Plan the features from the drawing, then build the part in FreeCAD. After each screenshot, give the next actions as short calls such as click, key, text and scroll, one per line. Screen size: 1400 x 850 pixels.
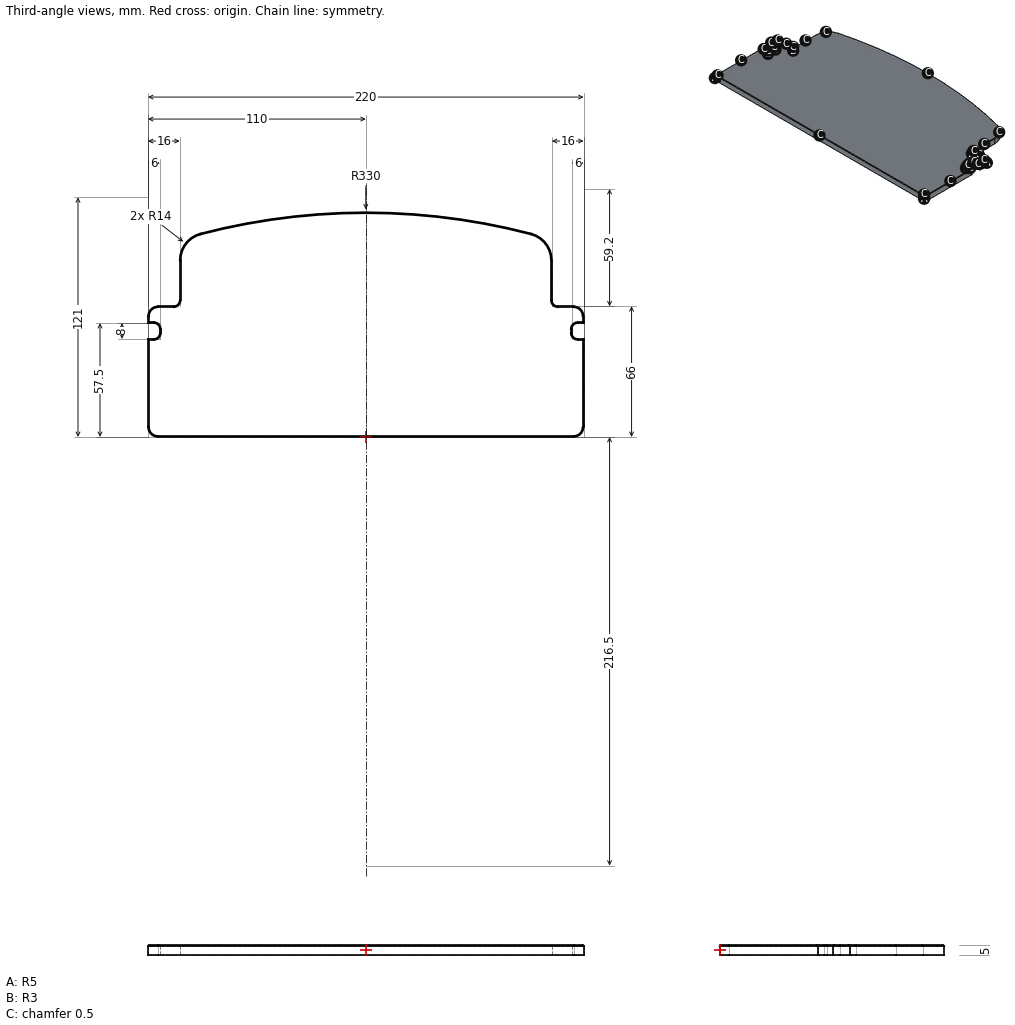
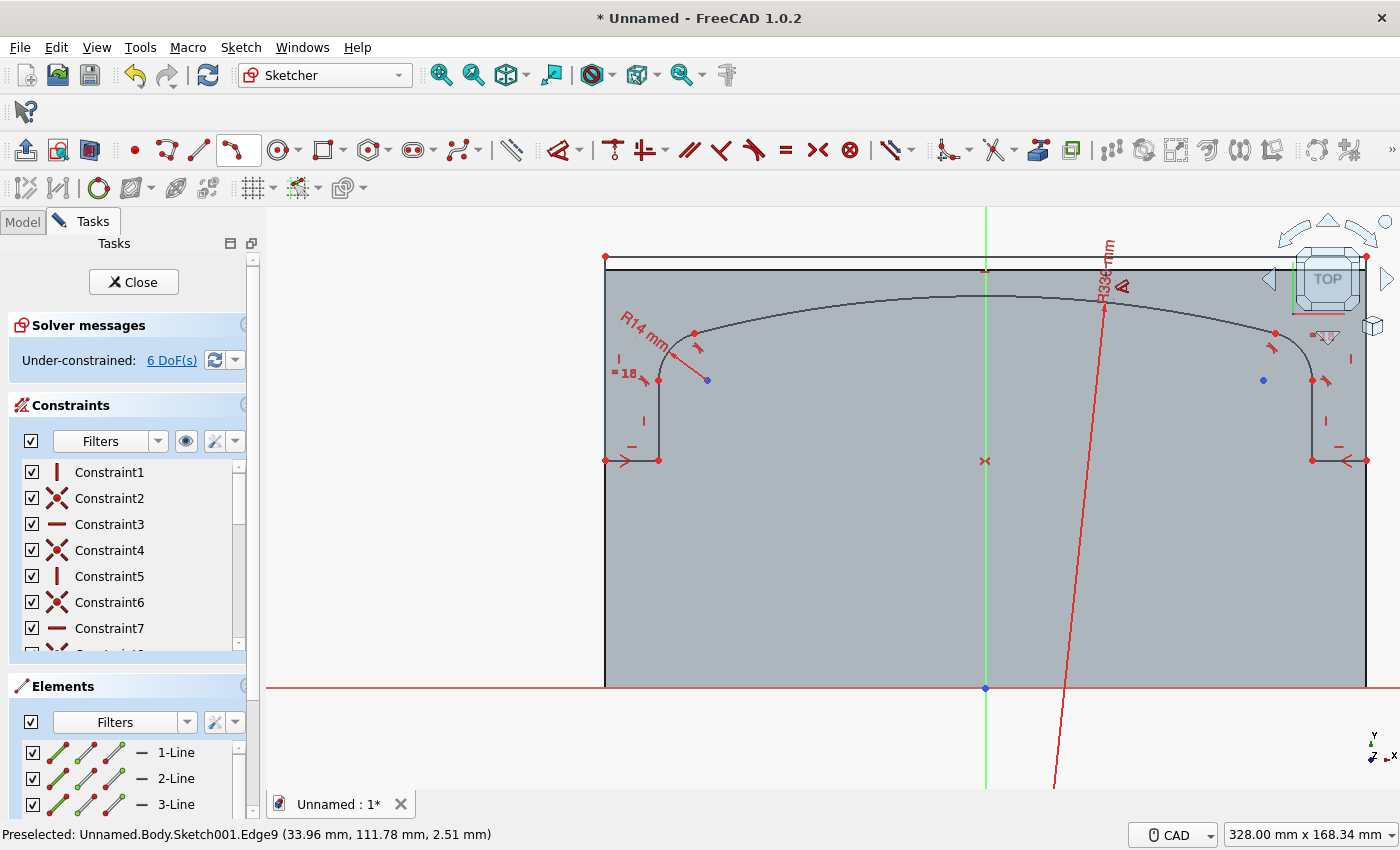
scroll(294, 617, down, 1)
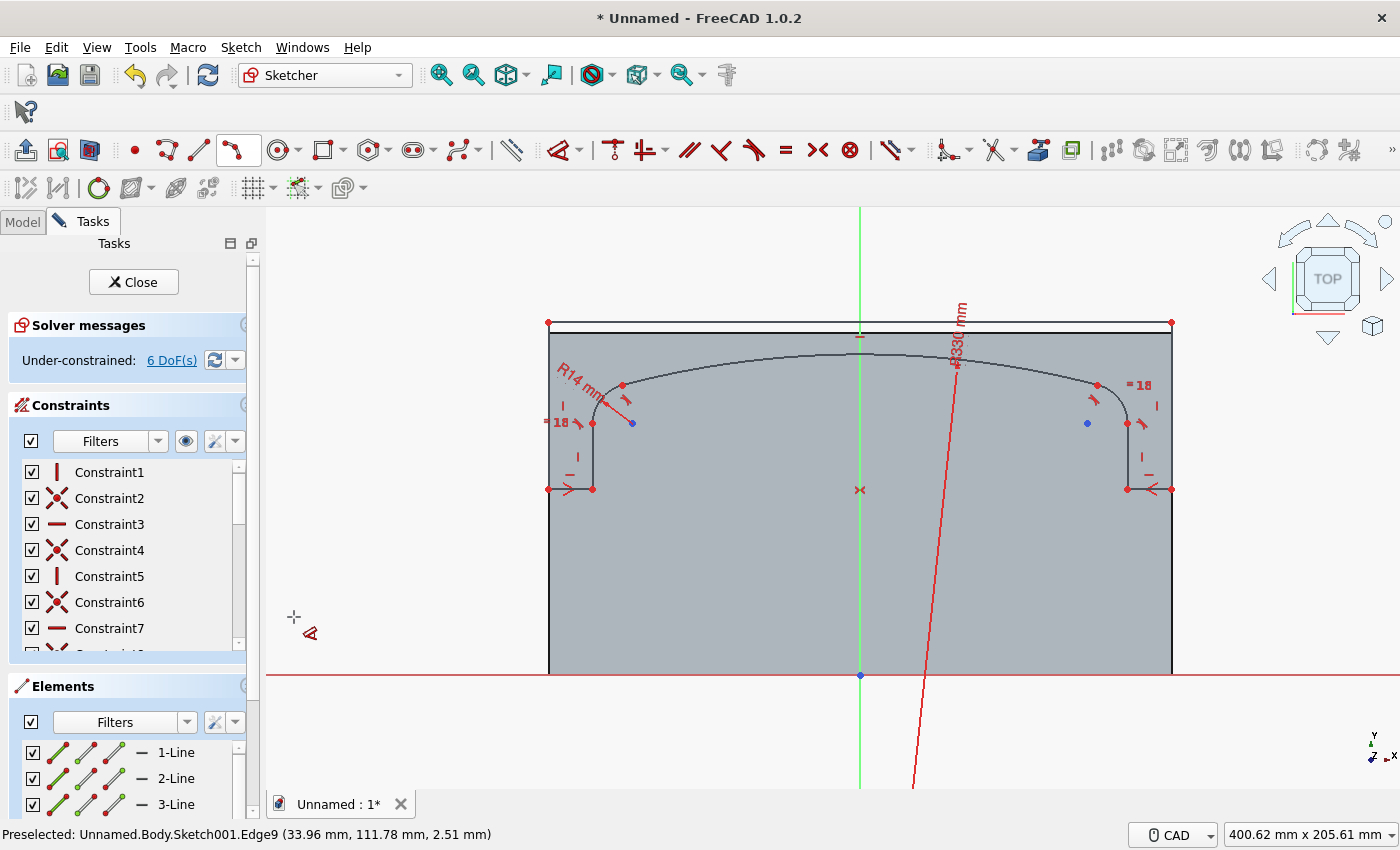
click(1141, 489)
click(1150, 455)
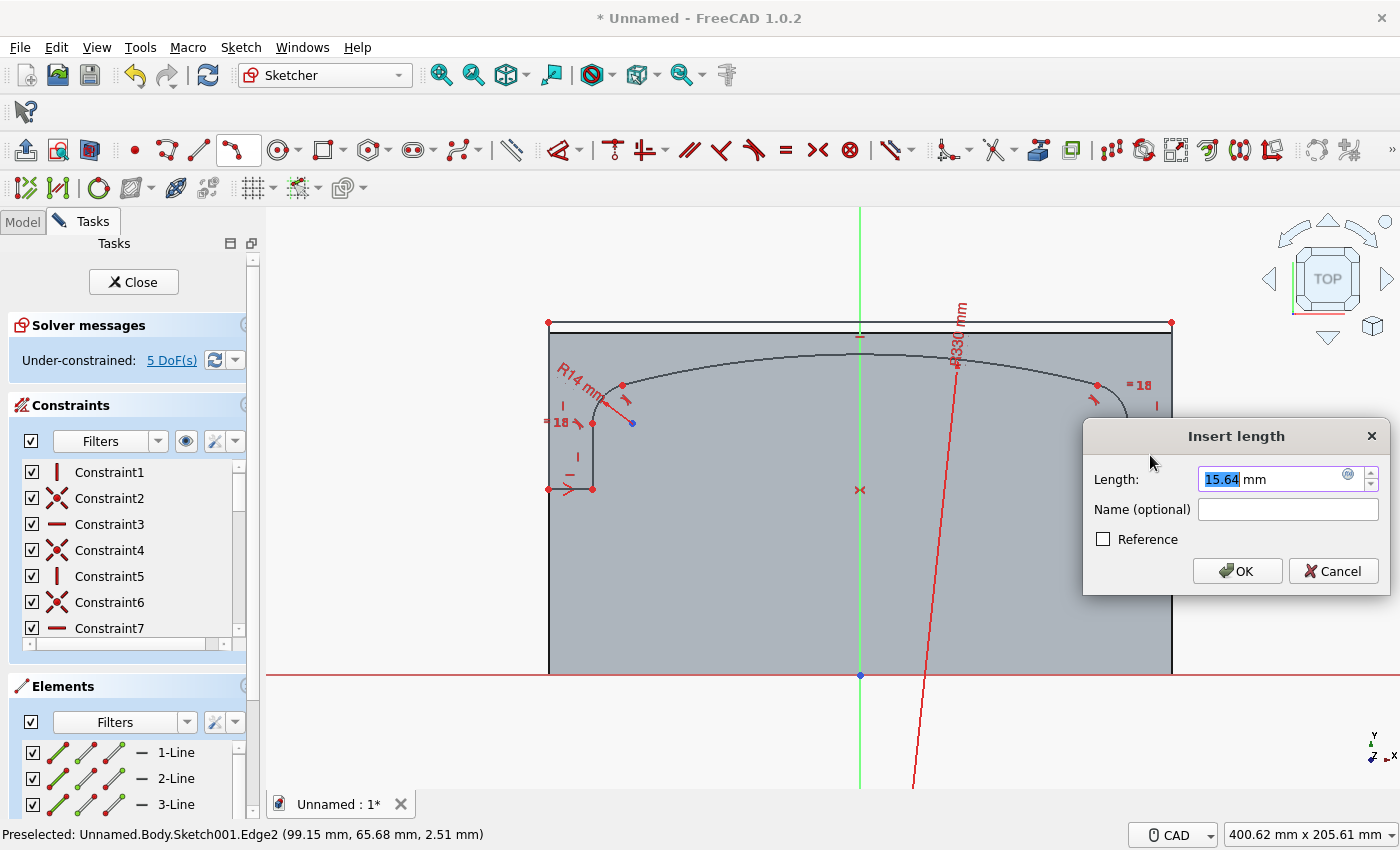
text(16)
key(Return)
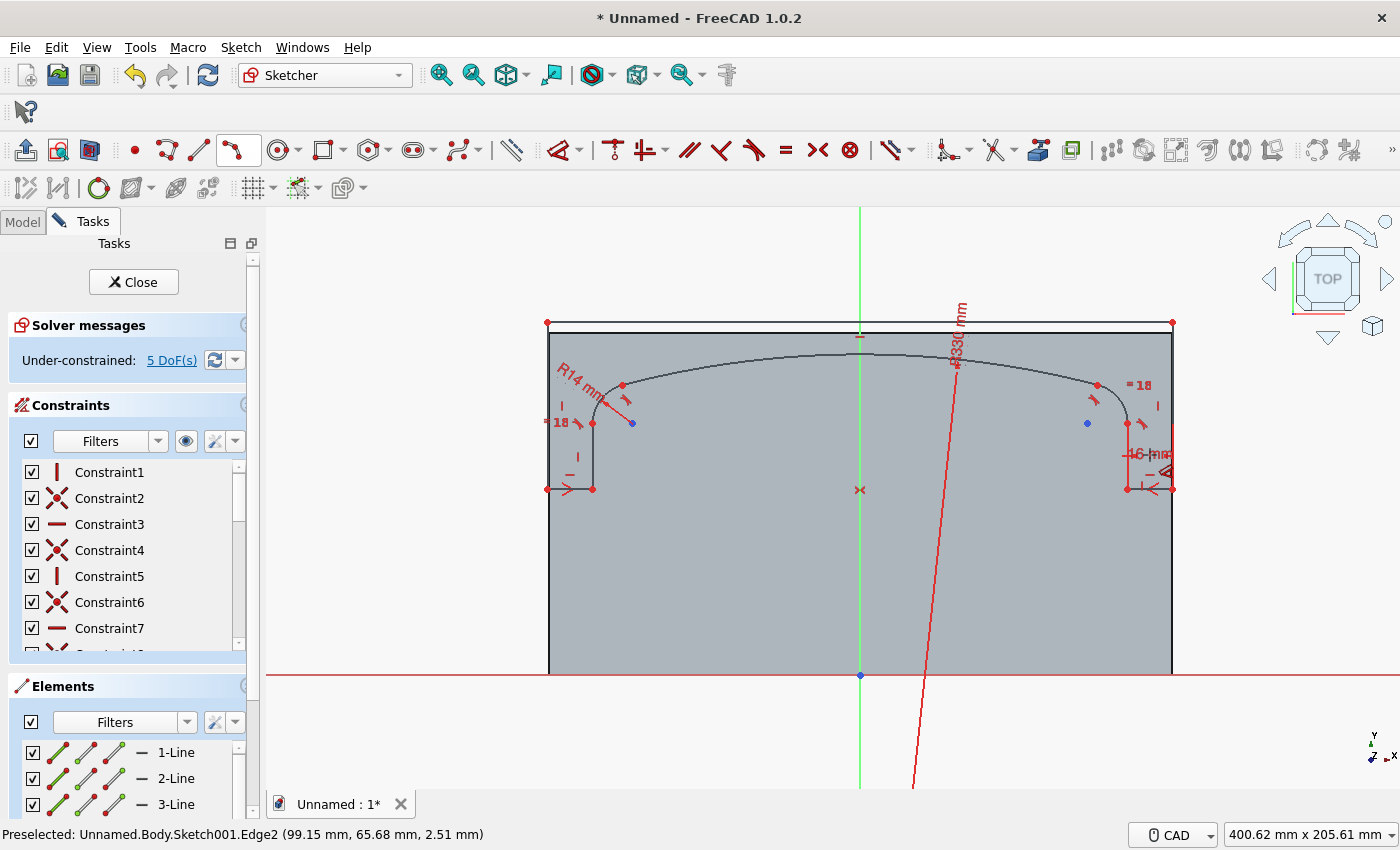
click(561, 489)
click(570, 455)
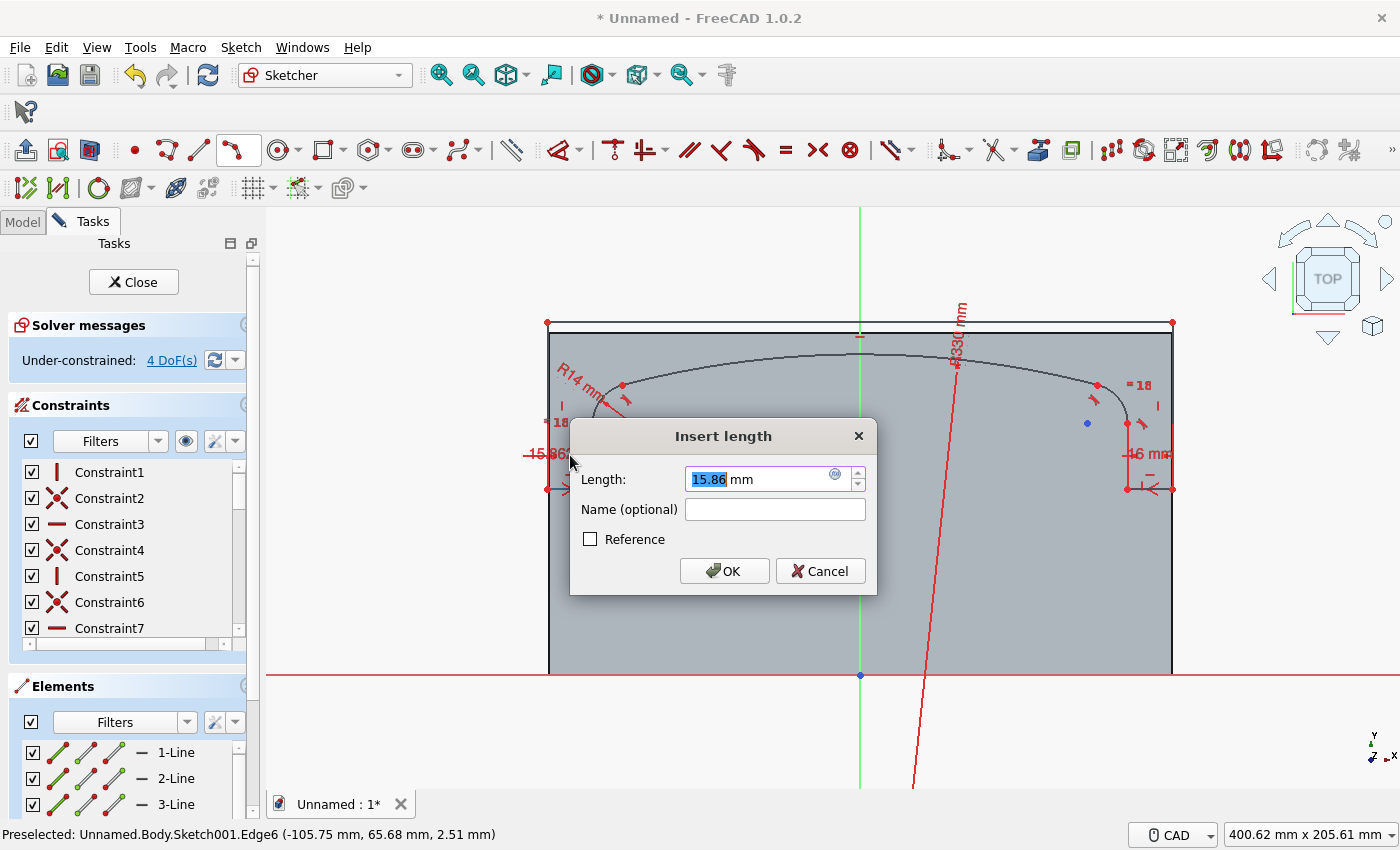
text(16)
key(Return)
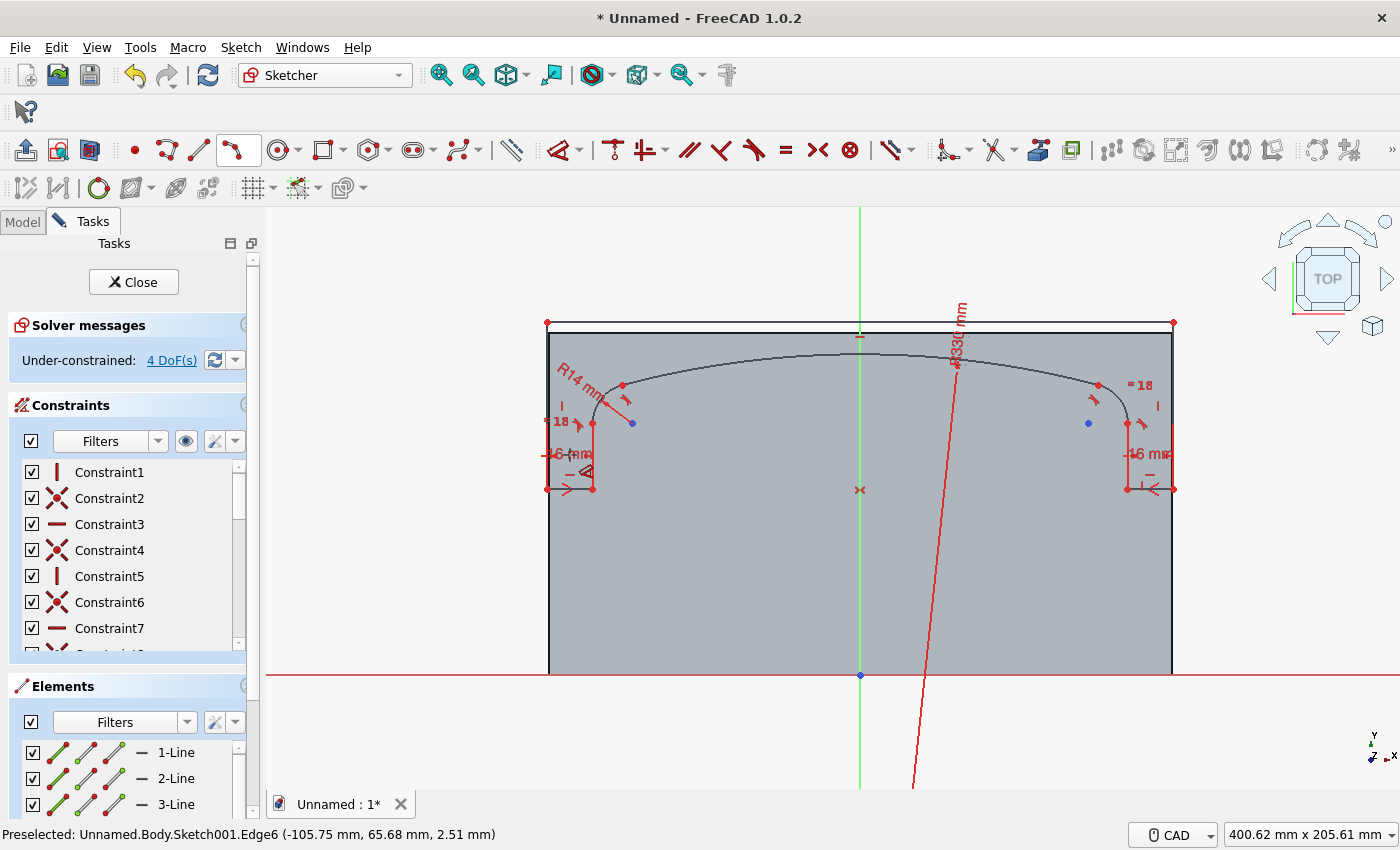
click(985, 322)
click(716, 288)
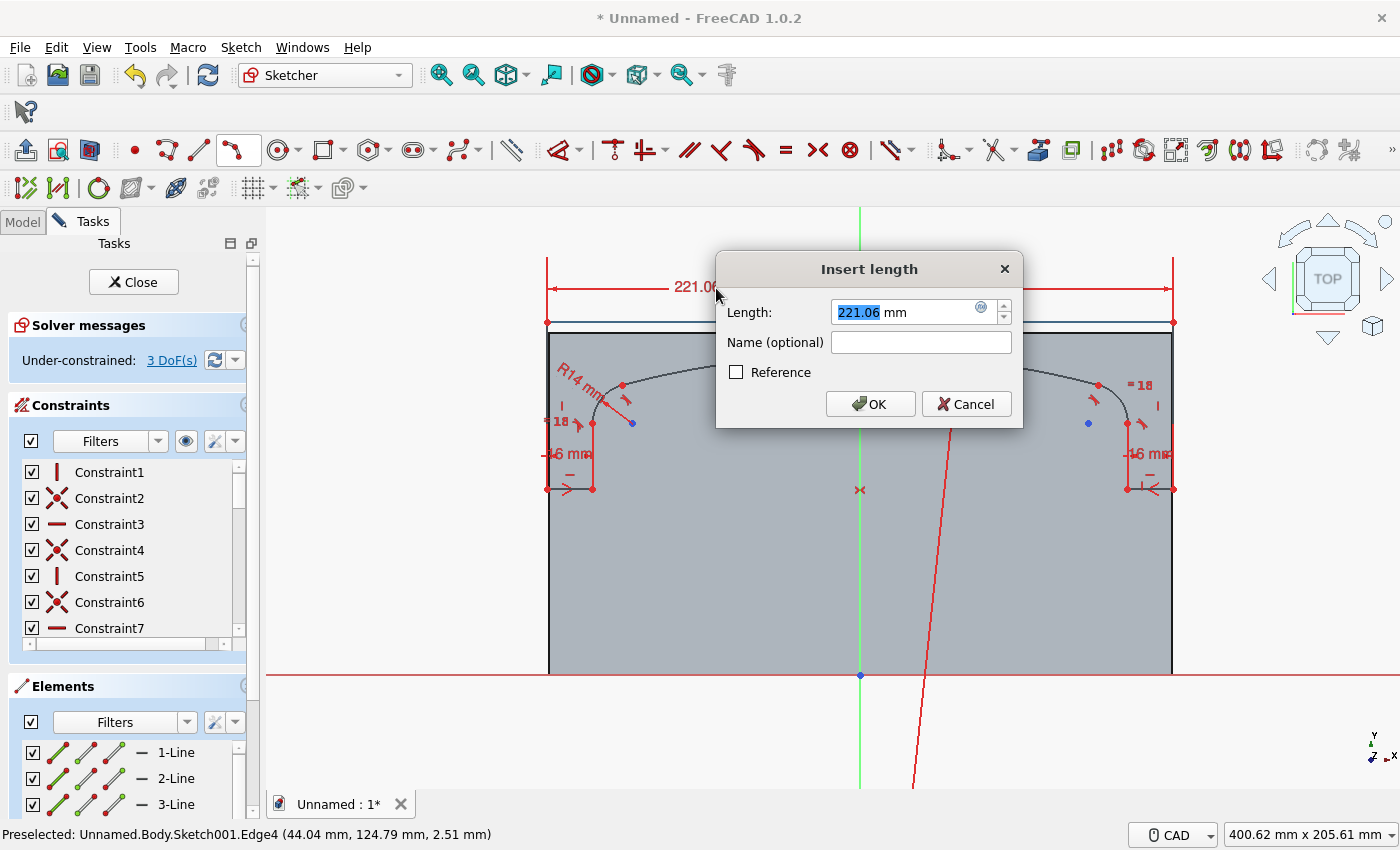
text(220)
key(Return)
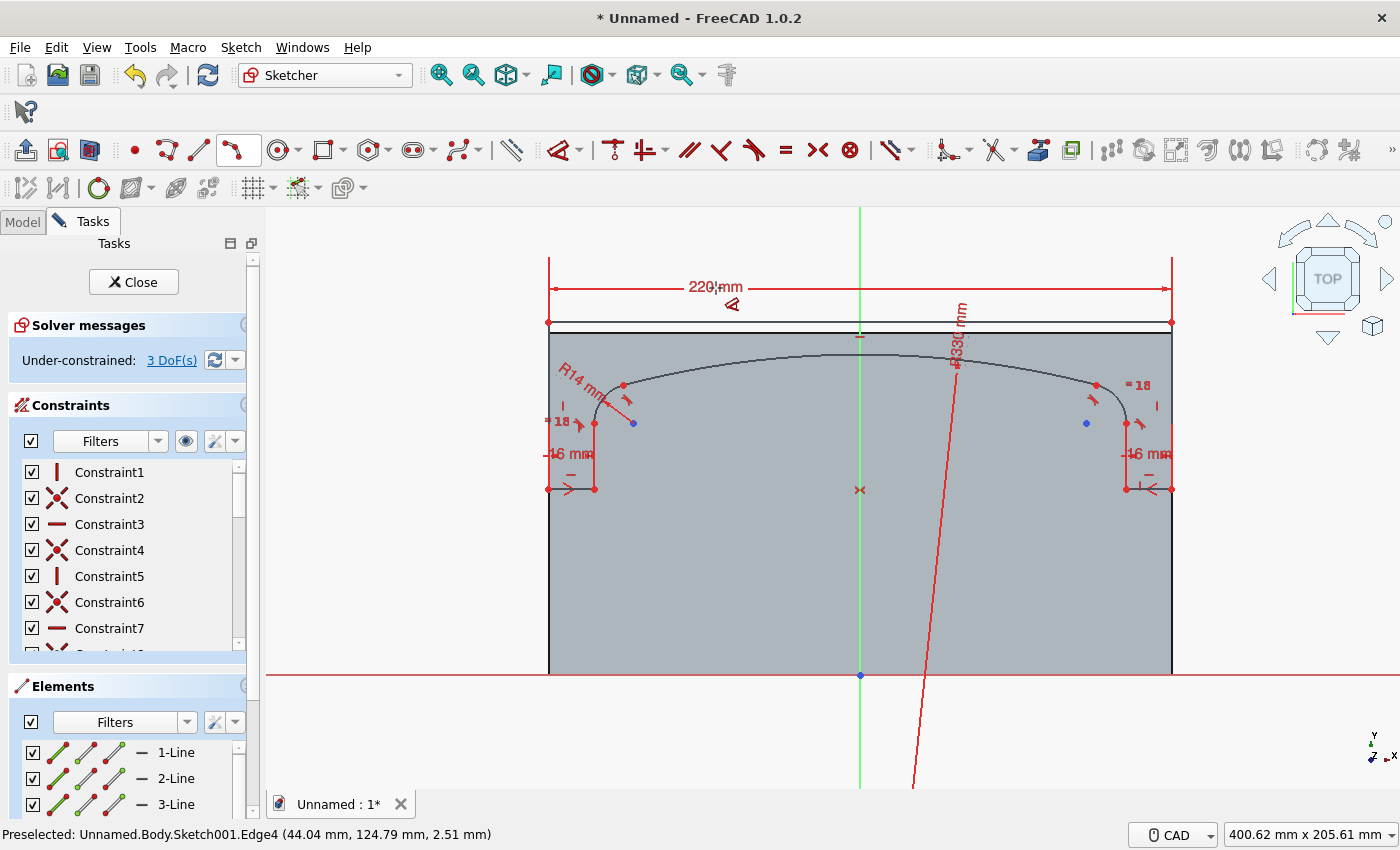
click(1126, 489)
click(1160, 582)